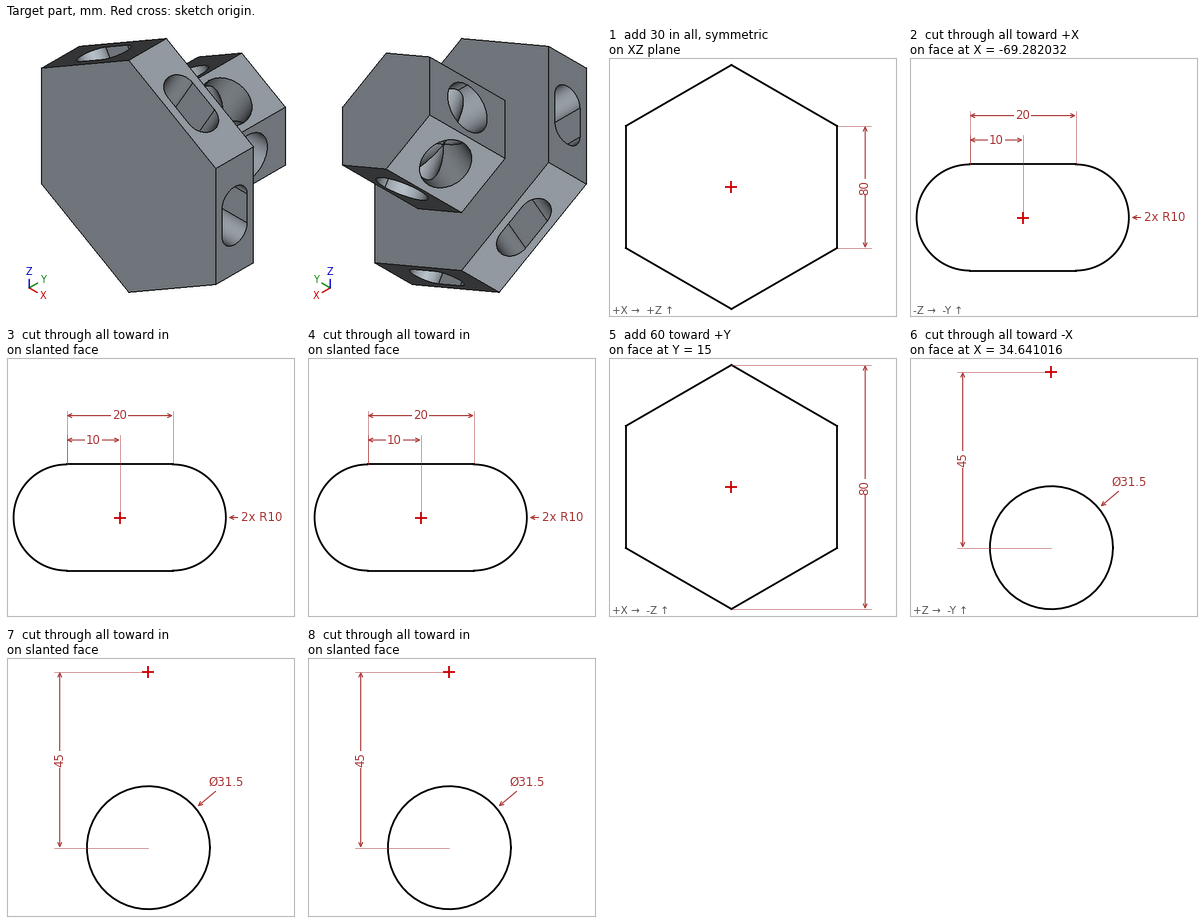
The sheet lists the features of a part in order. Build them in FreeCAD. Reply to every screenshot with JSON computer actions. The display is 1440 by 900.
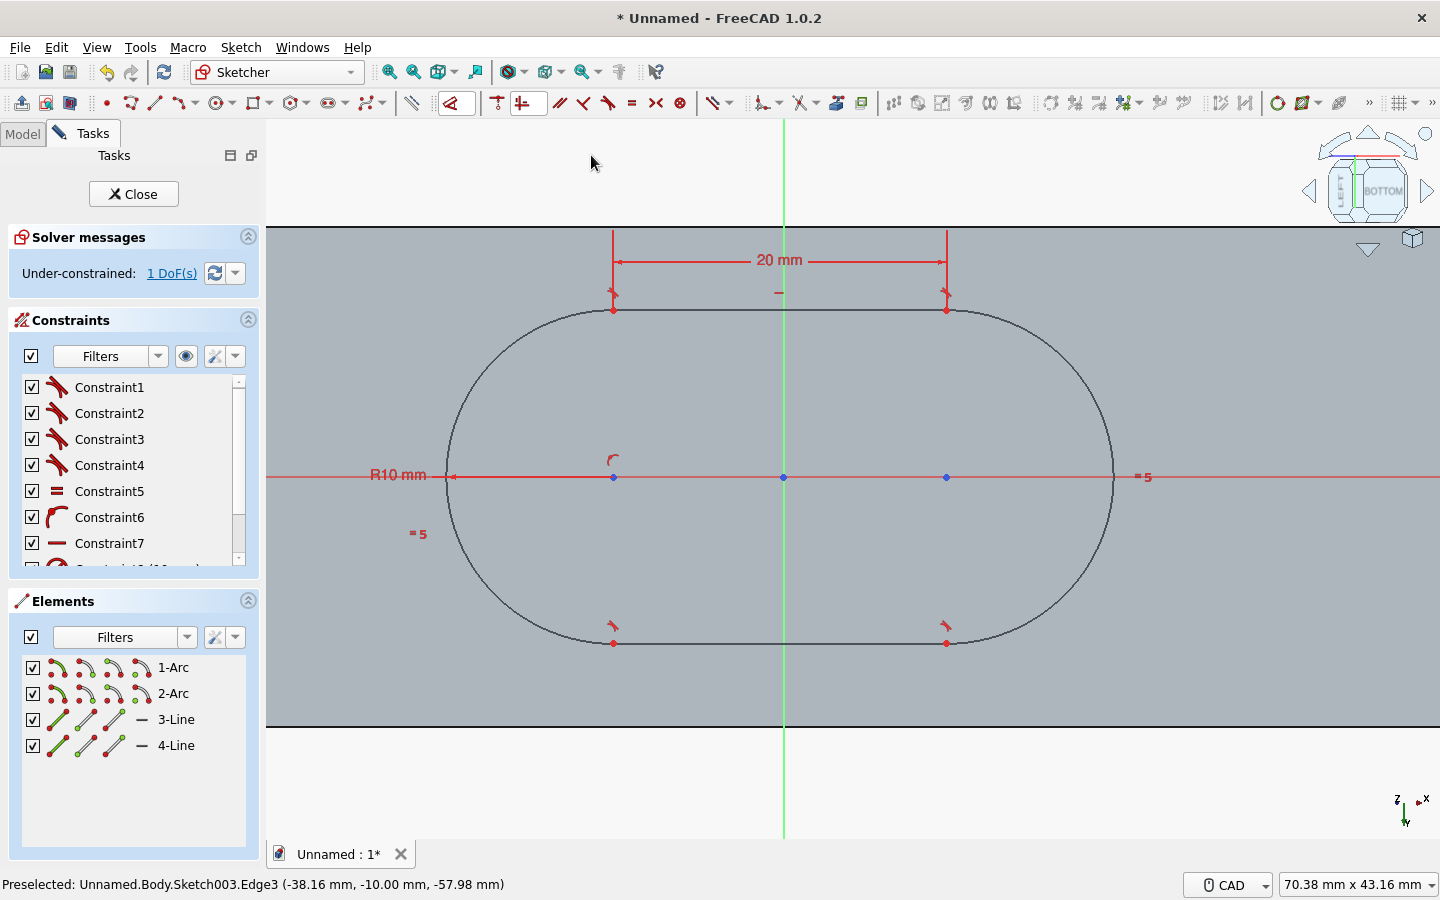
{"action": "left_click", "coordinate": [613, 310]}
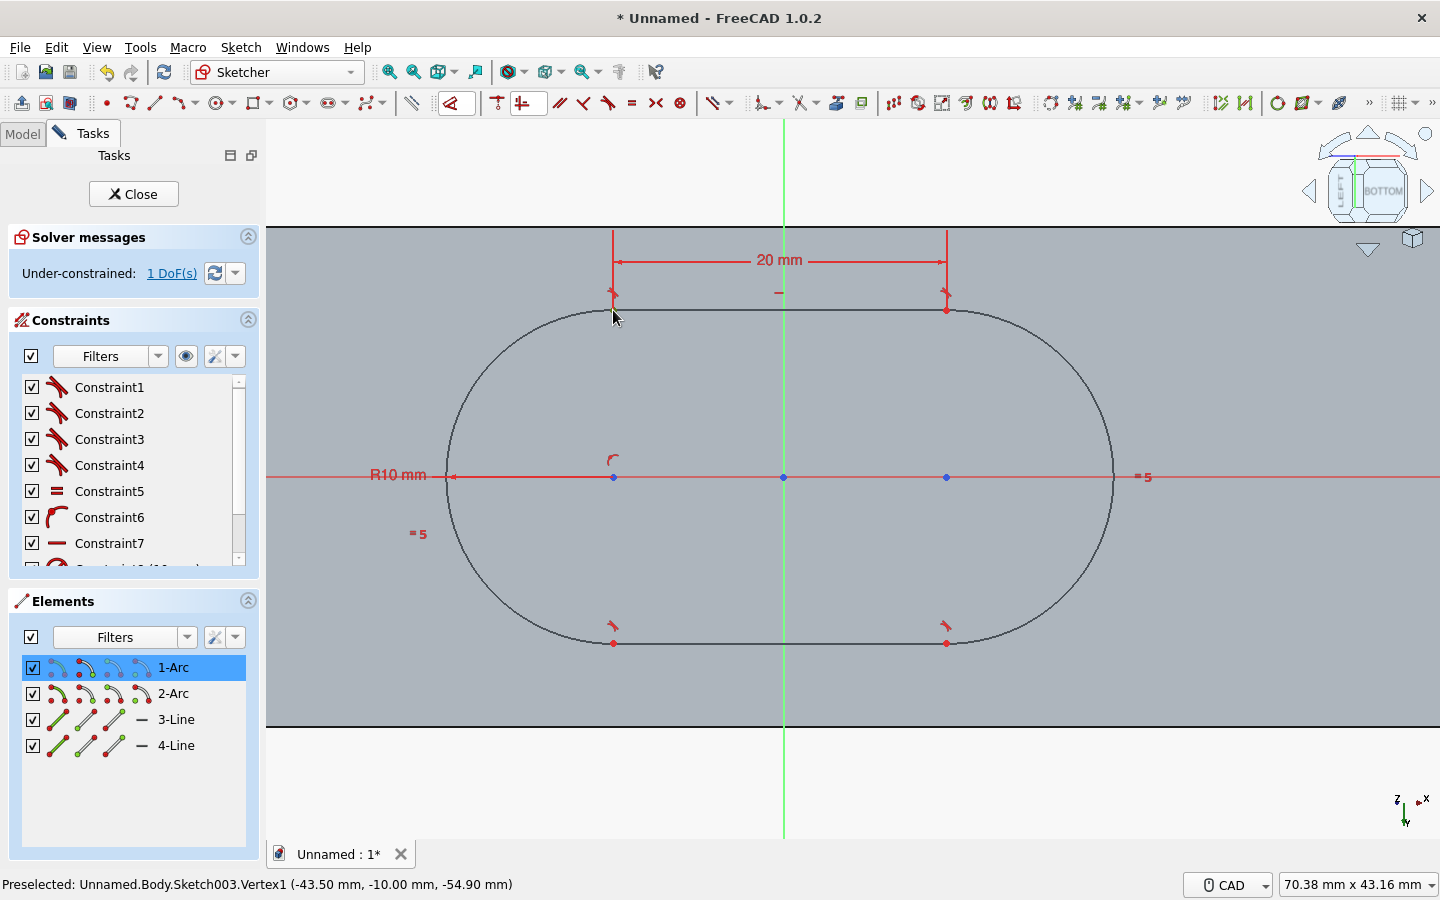
{"action": "left_click", "coordinate": [470, 104]}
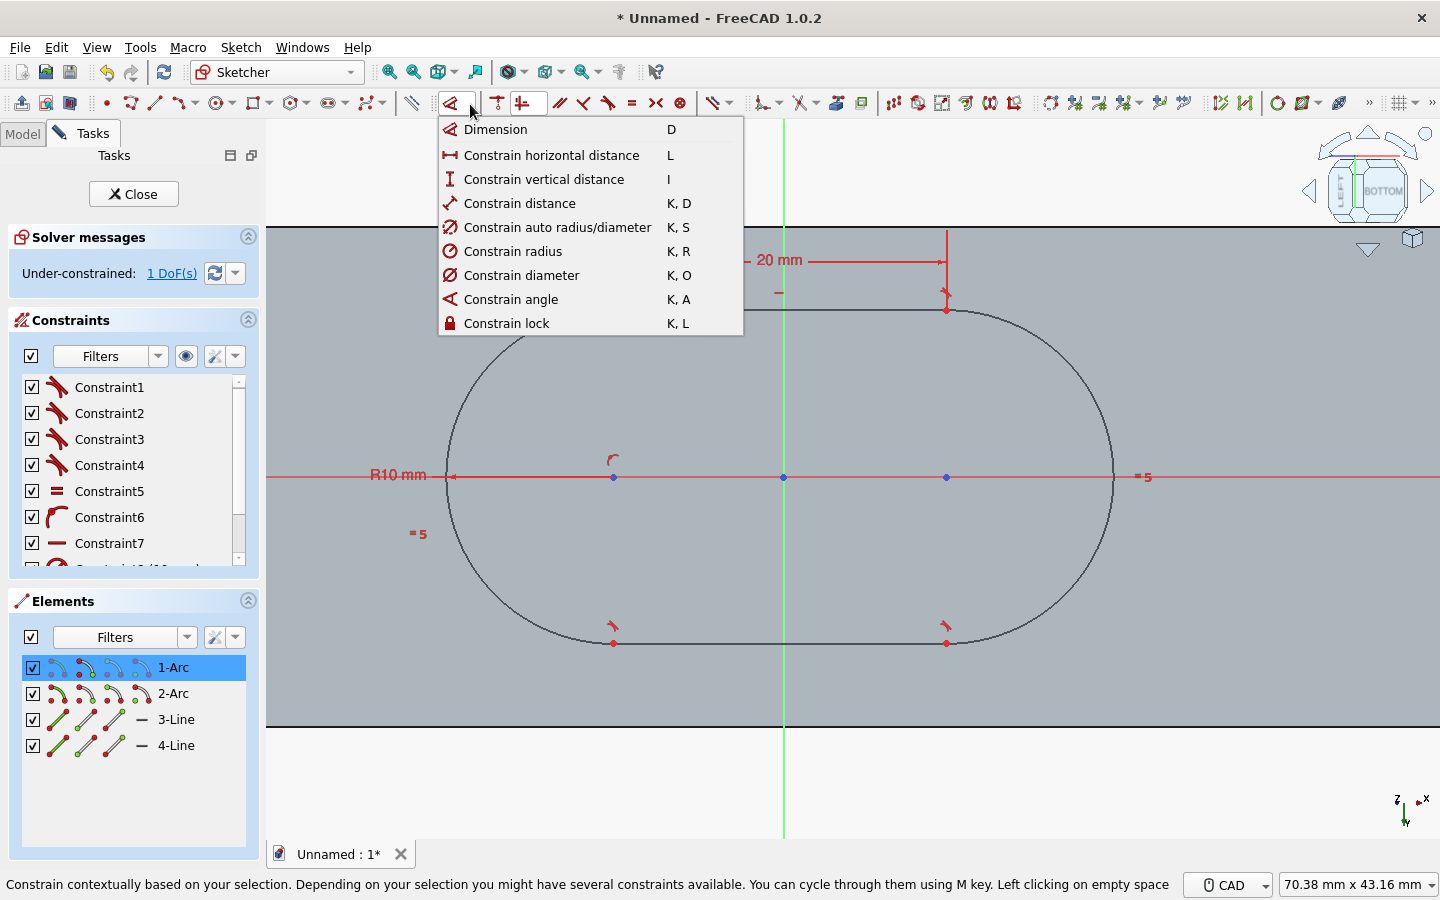
{"action": "left_click", "coordinate": [591, 155]}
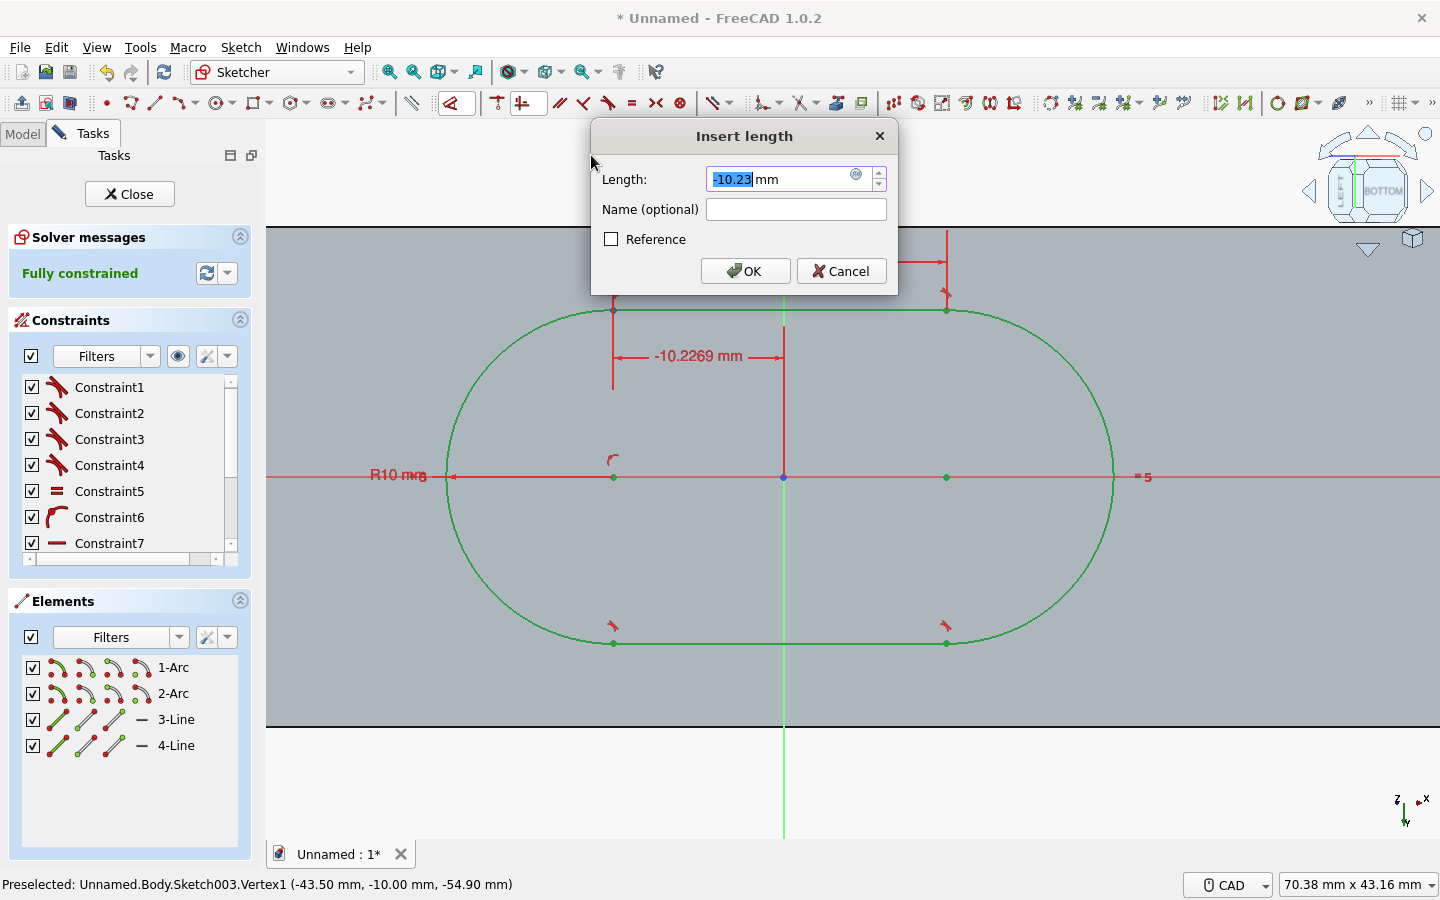
{"action": "type", "text": "-10"}
{"action": "key", "text": "Return"}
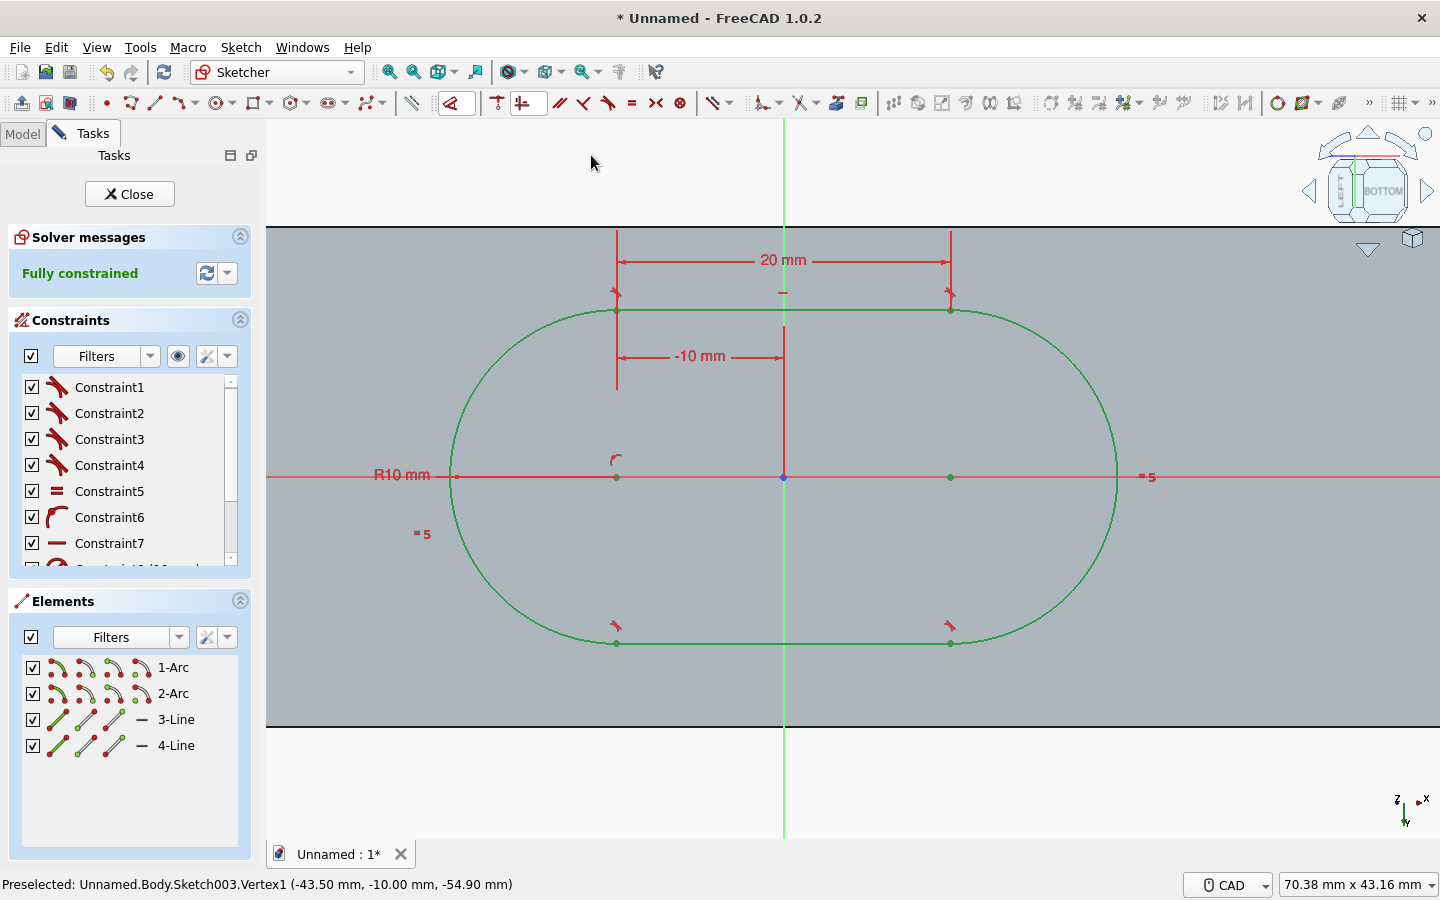
{"action": "left_click", "coordinate": [130, 194]}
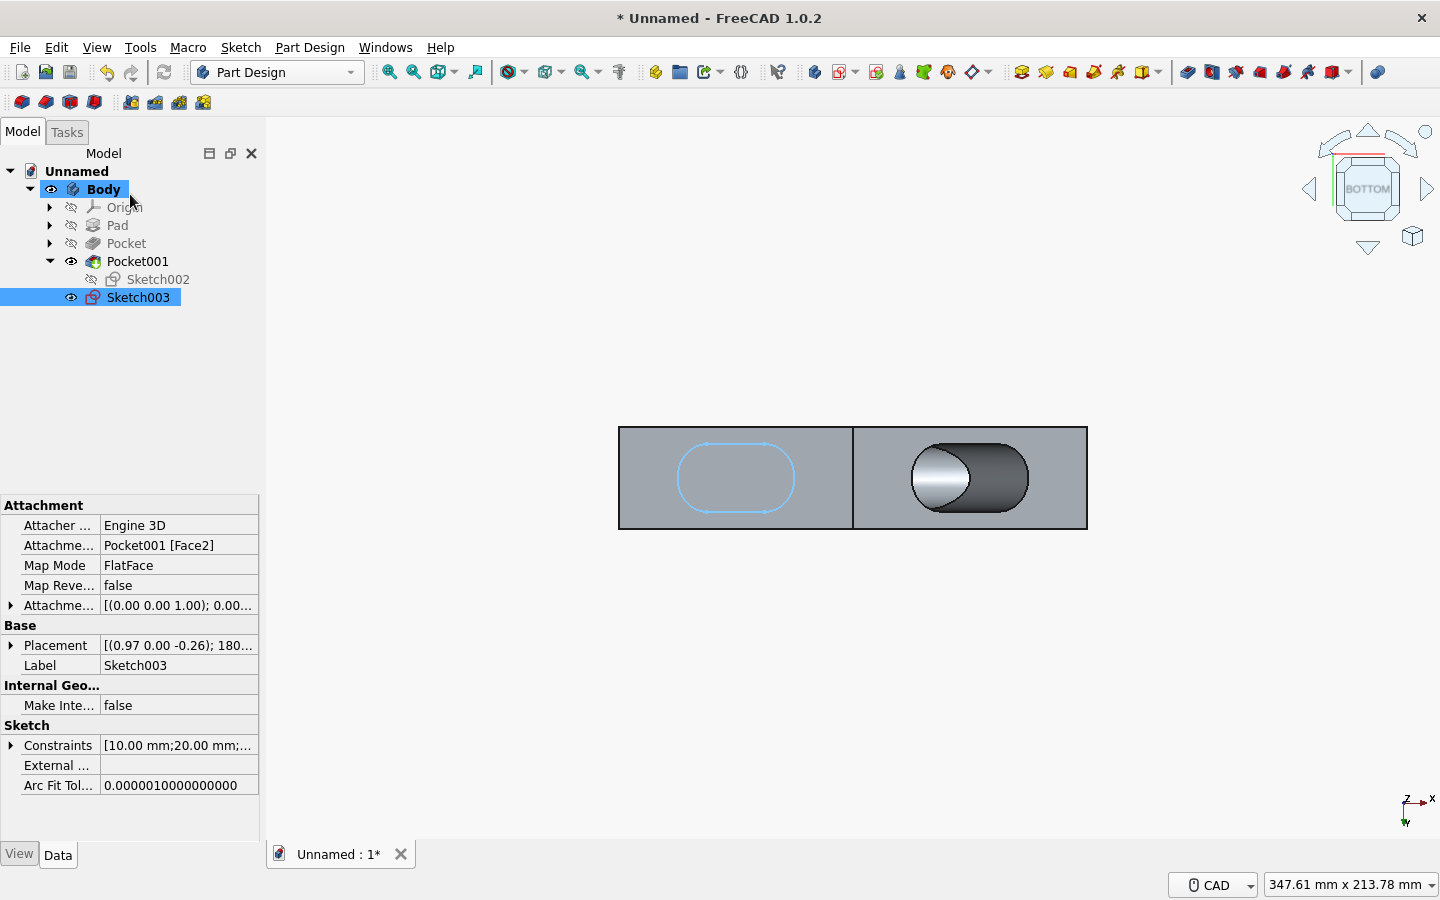
{"action": "left_click", "coordinate": [1188, 72]}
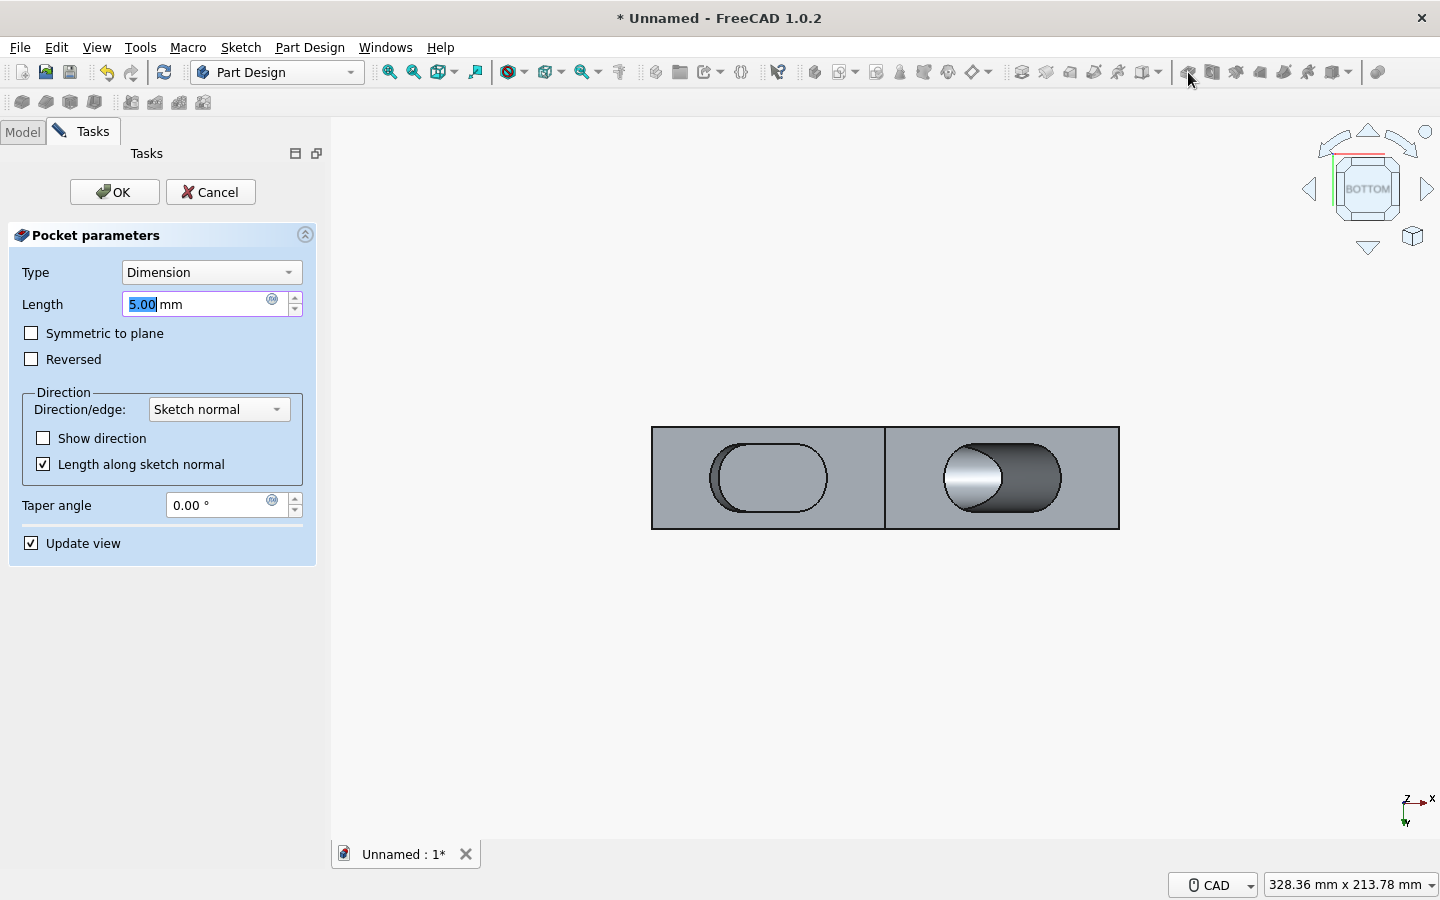
{"action": "left_click", "coordinate": [212, 272]}